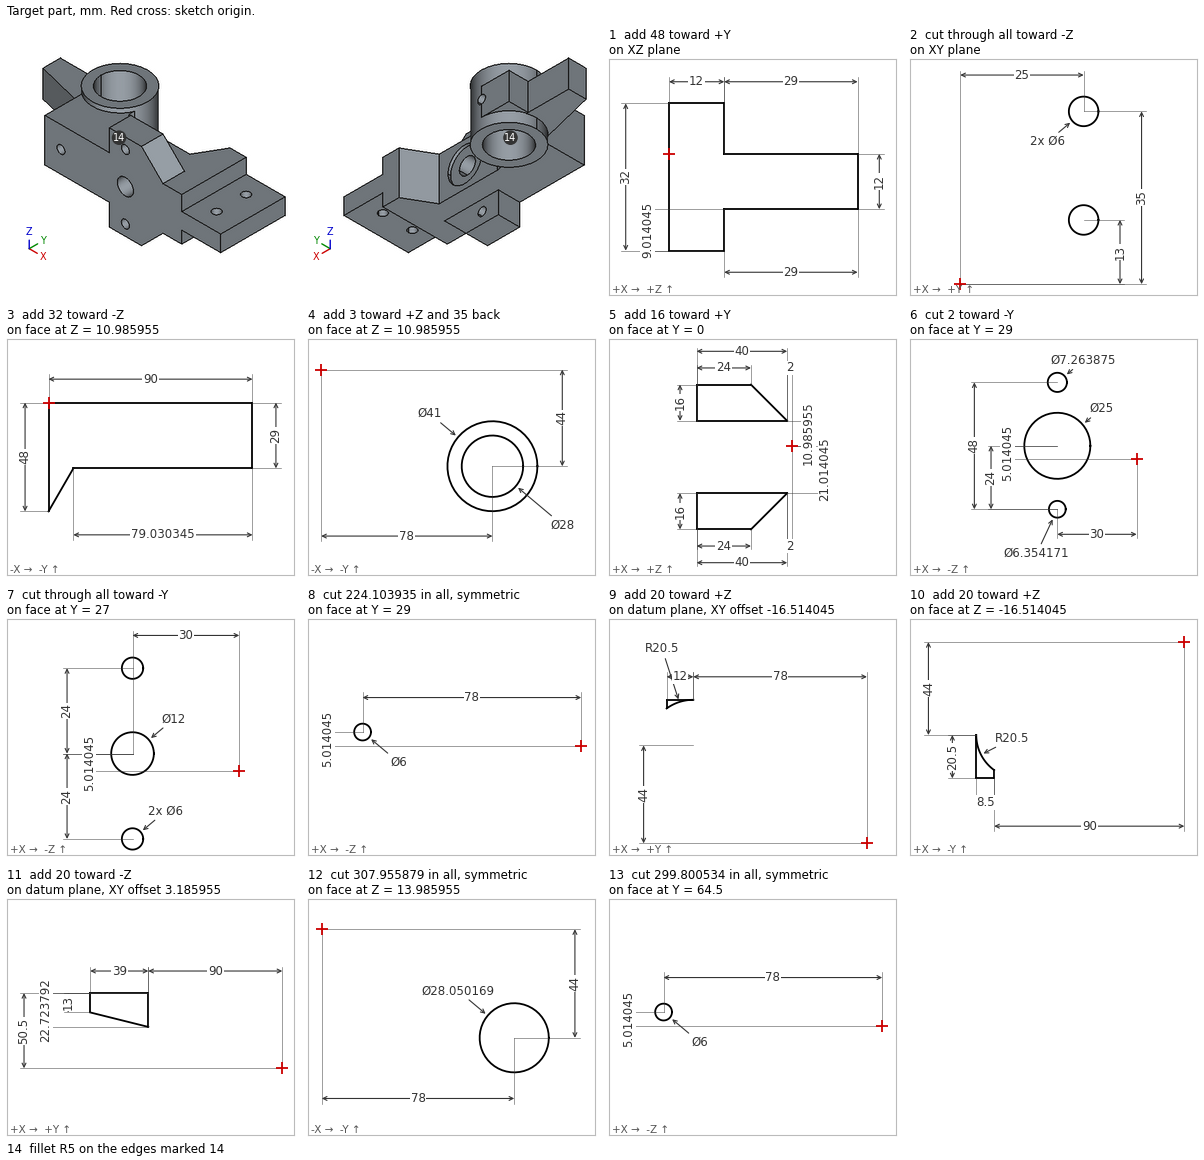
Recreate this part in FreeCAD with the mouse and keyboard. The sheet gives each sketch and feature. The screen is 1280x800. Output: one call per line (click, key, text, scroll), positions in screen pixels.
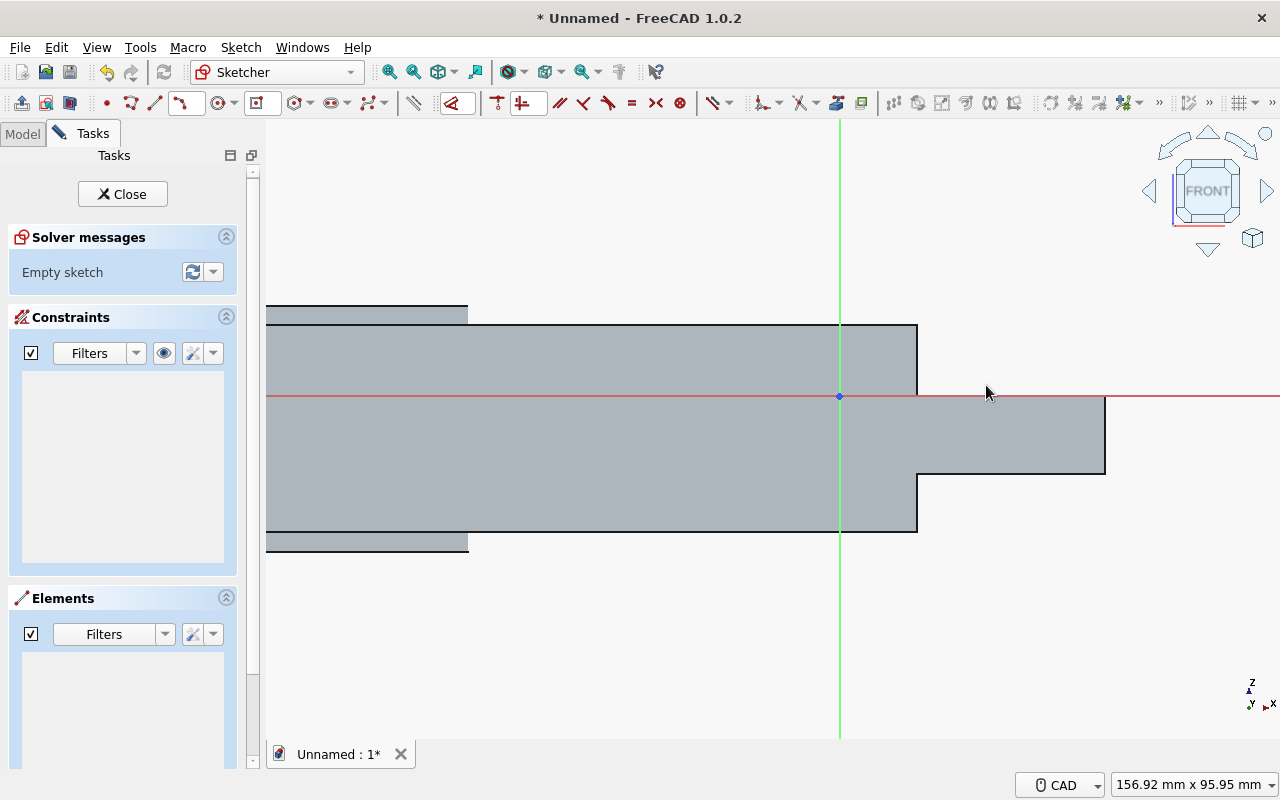
click(132, 104)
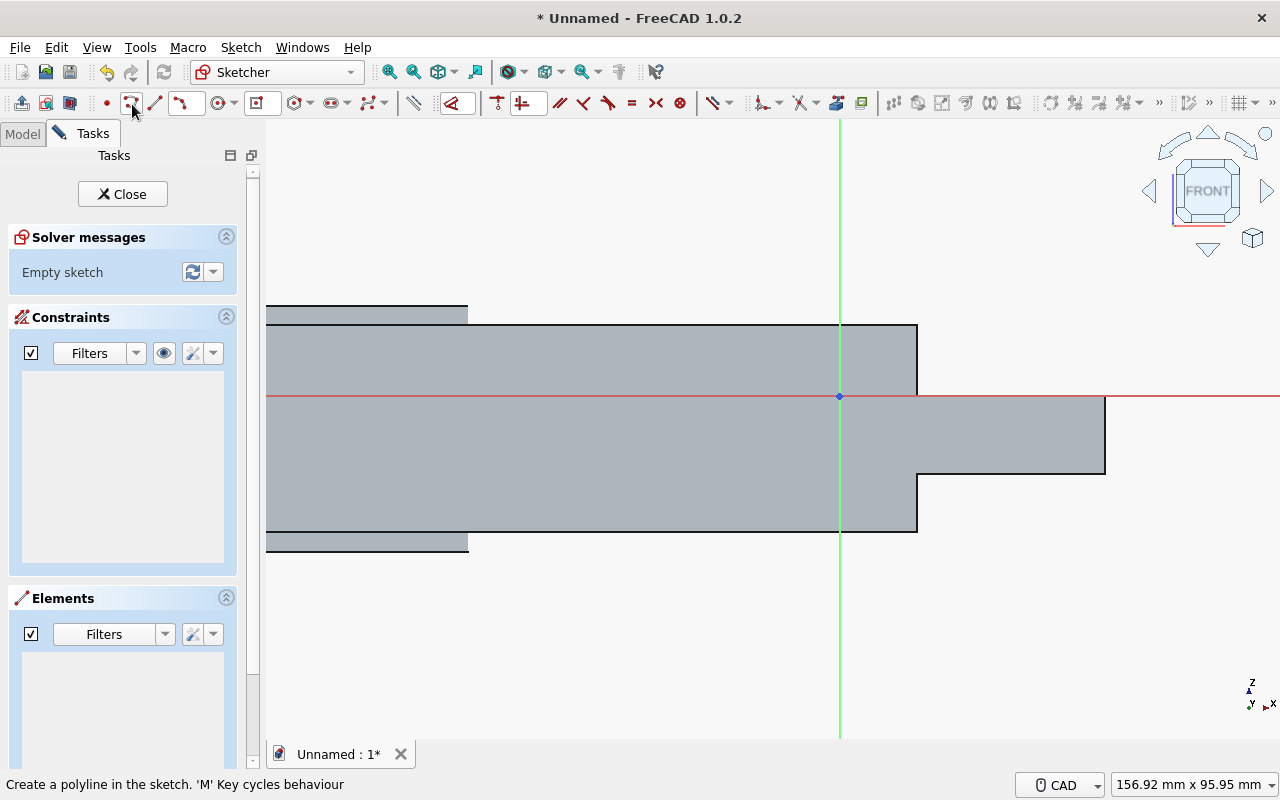
scroll(827, 532, up, 2)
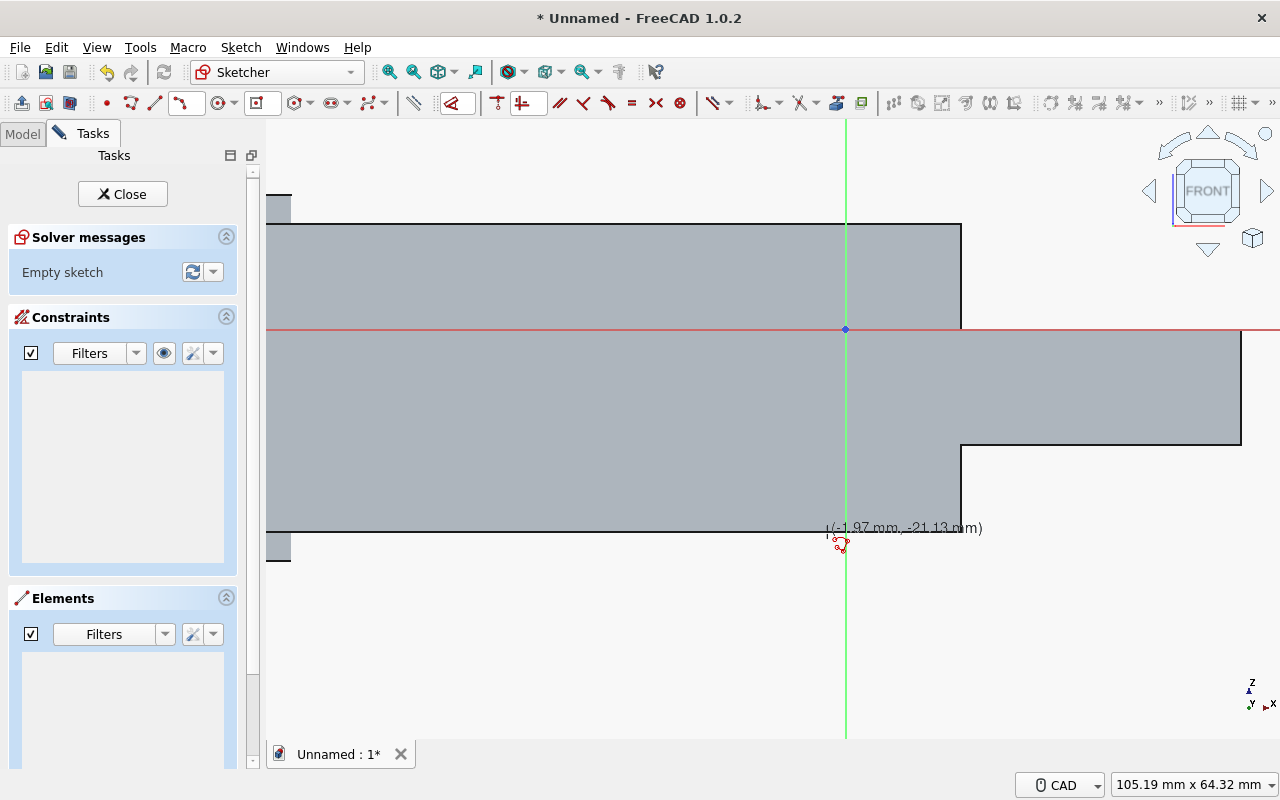
click(826, 532)
click(441, 532)
click(441, 686)
click(672, 686)
click(826, 533)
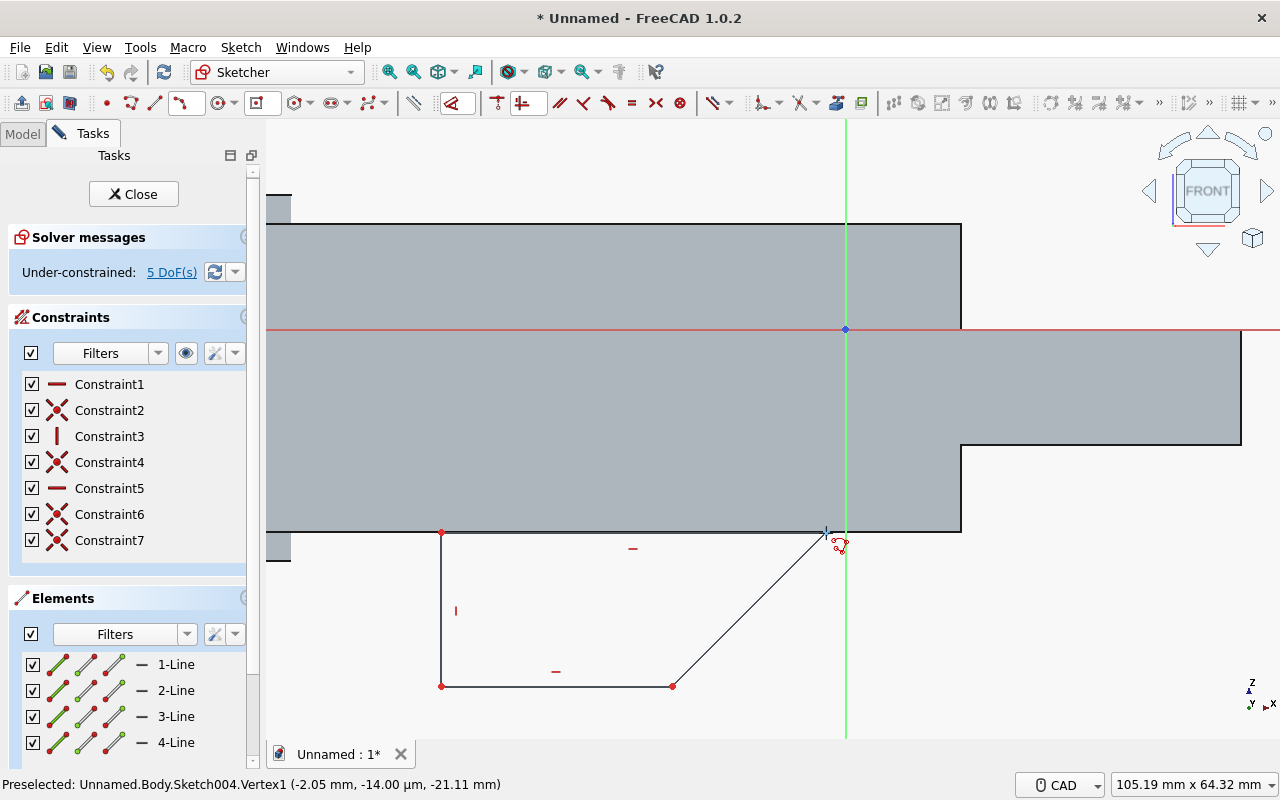
click(826, 224)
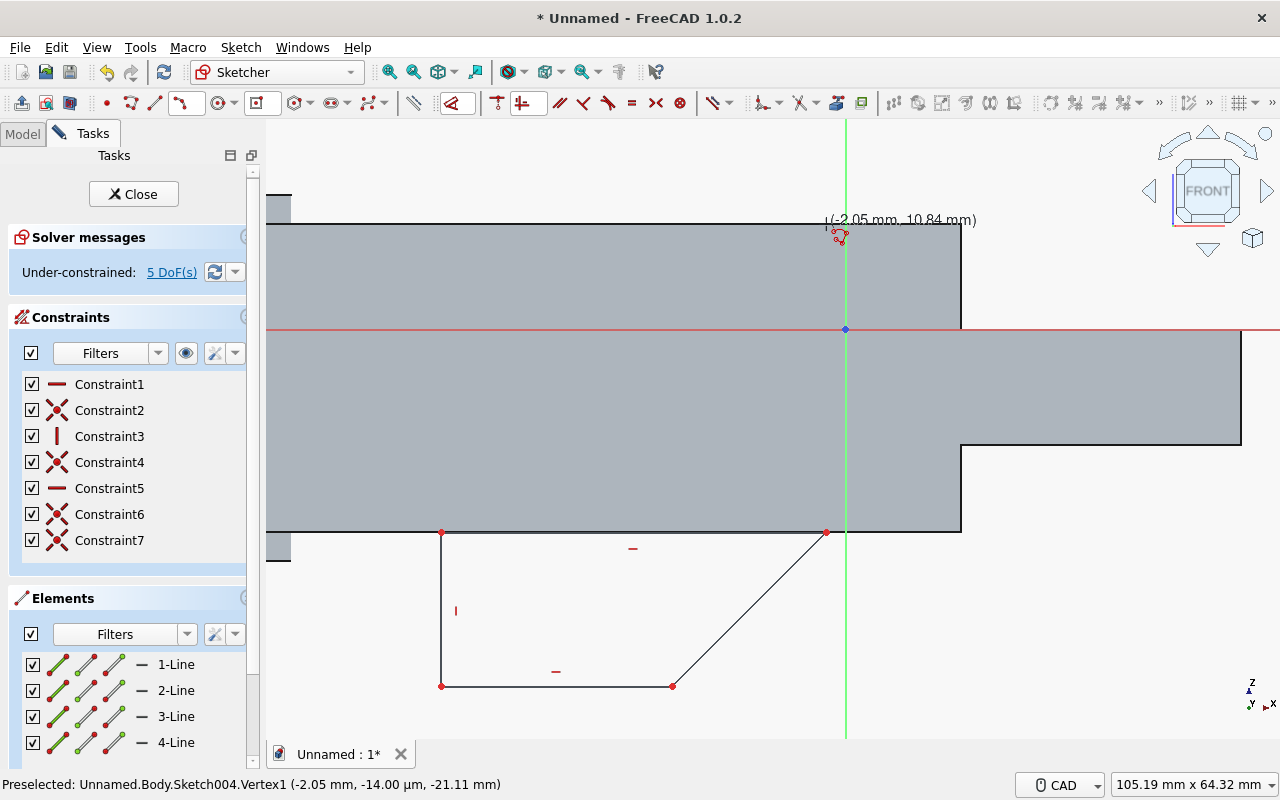
scroll(829, 533, down, 2)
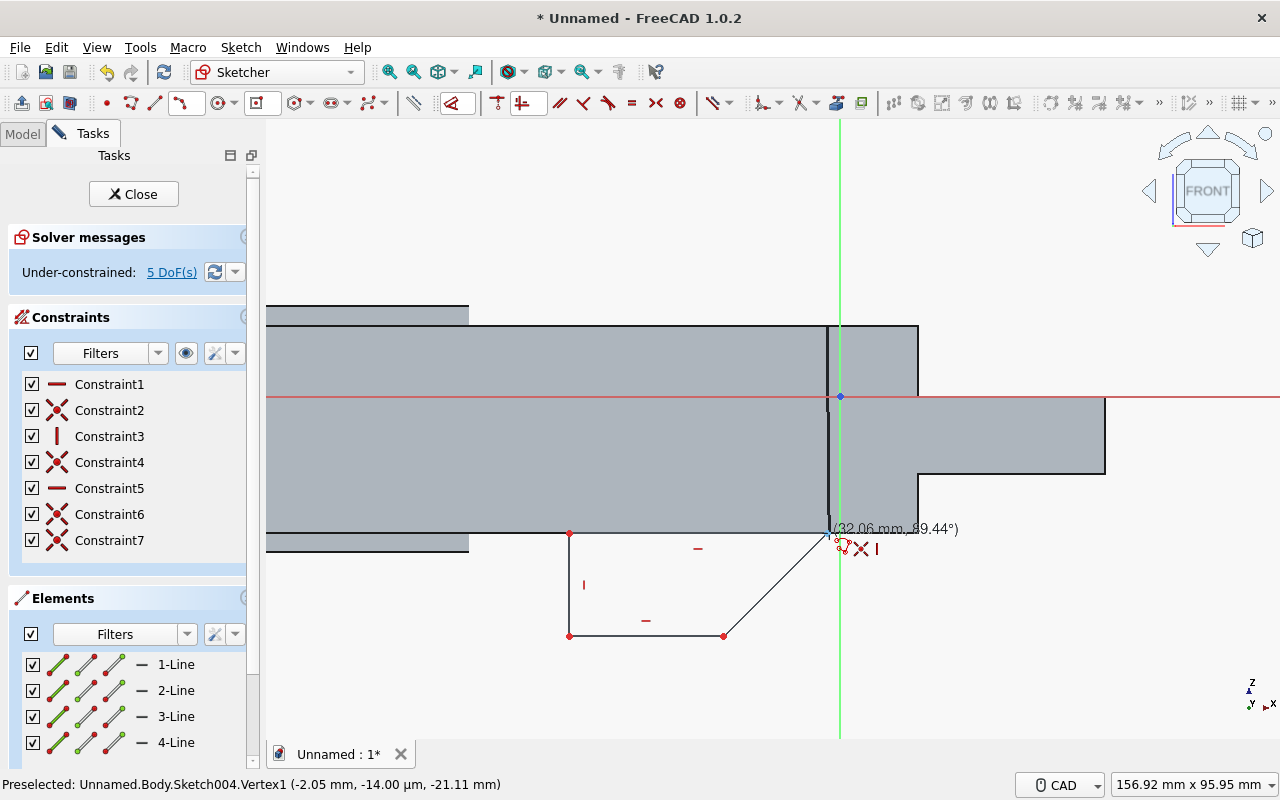
click(724, 222)
click(569, 222)
click(569, 326)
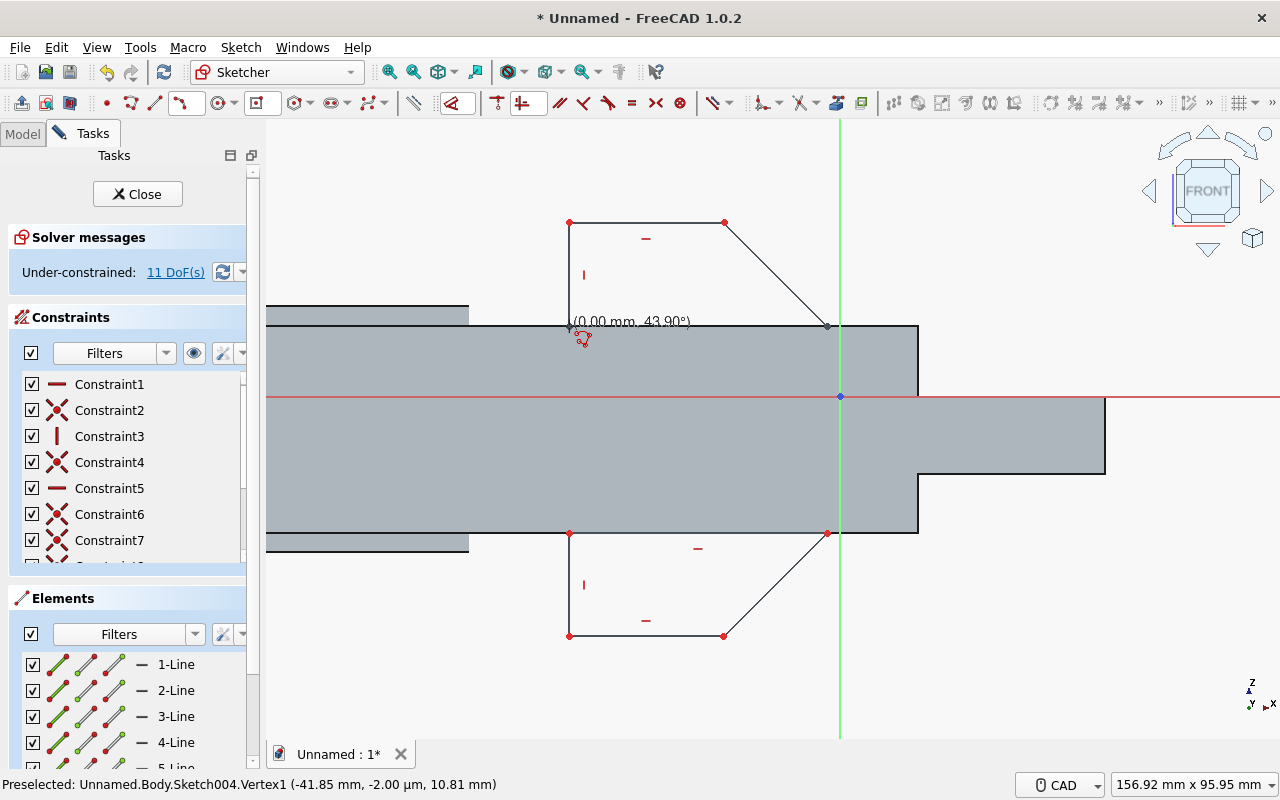
scroll(827, 326, up, 2)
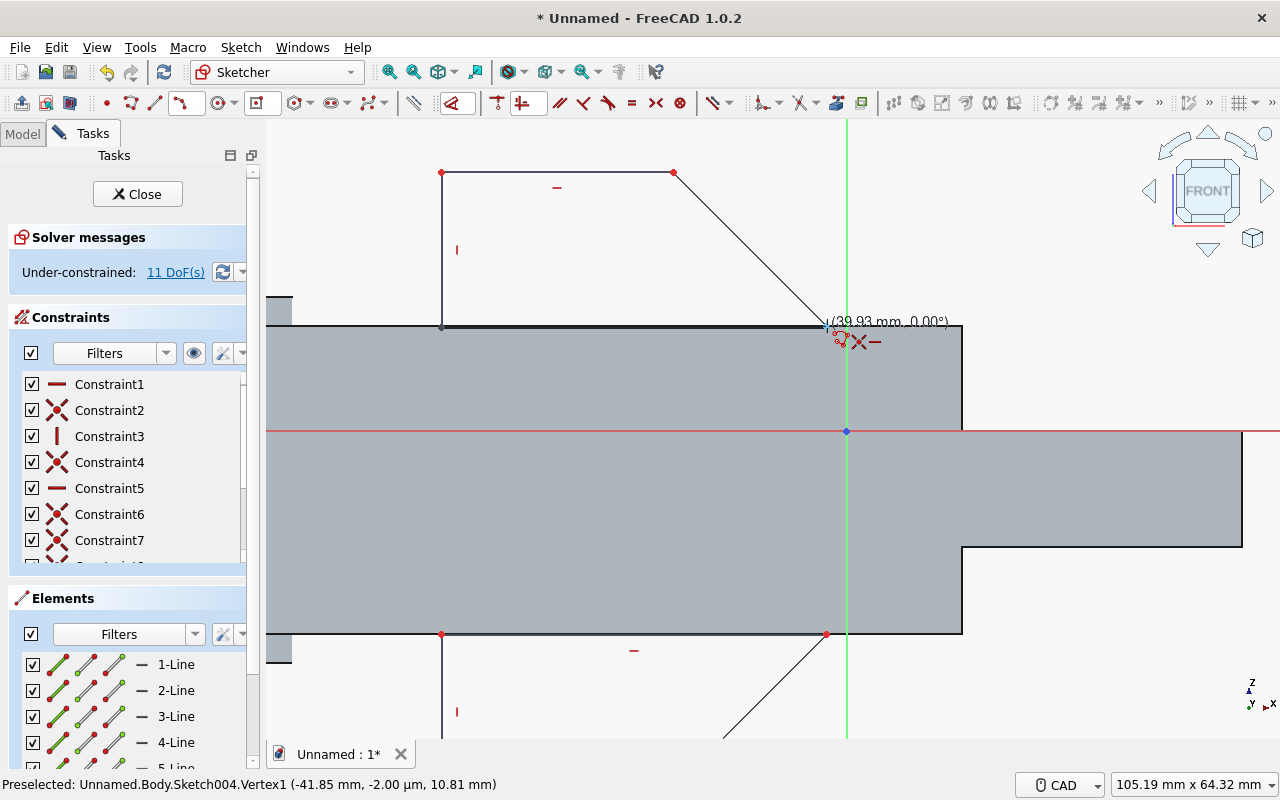
click(827, 327)
key(Escape)
key(Escape)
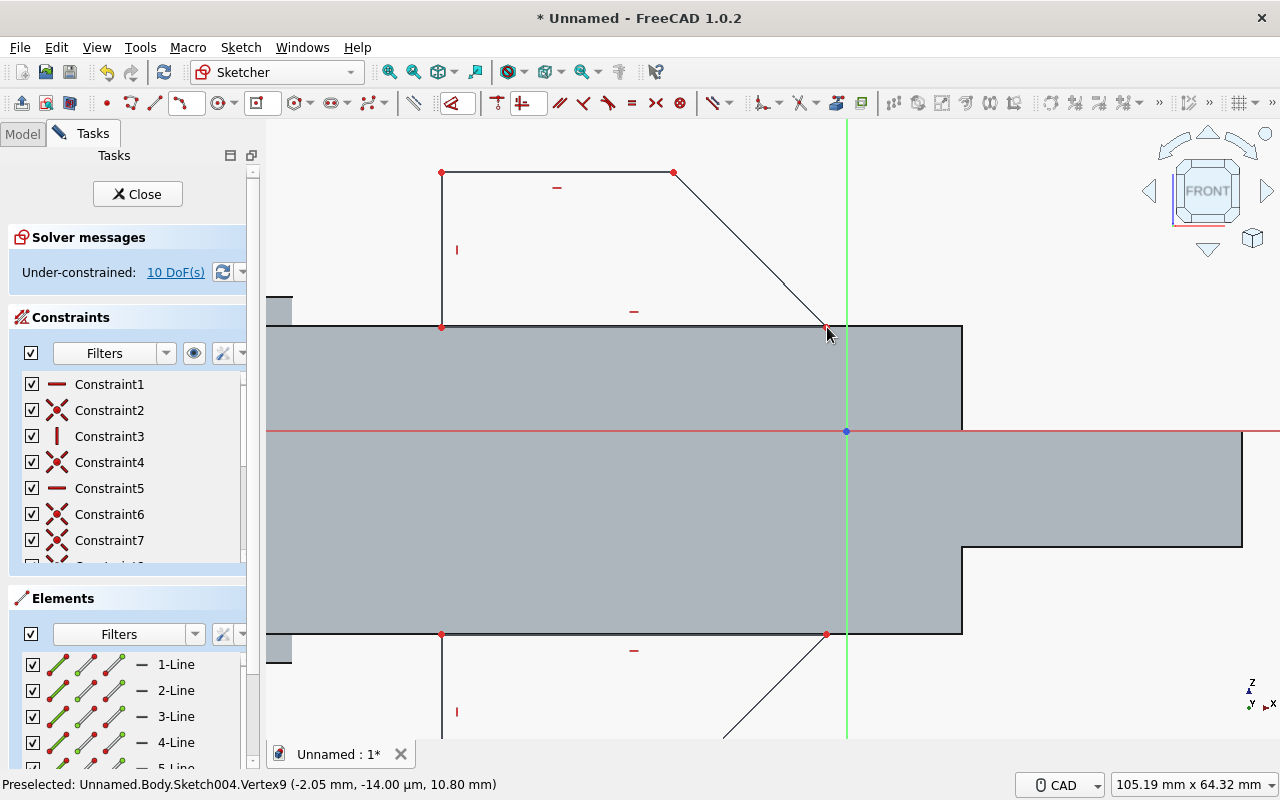
click(711, 635)